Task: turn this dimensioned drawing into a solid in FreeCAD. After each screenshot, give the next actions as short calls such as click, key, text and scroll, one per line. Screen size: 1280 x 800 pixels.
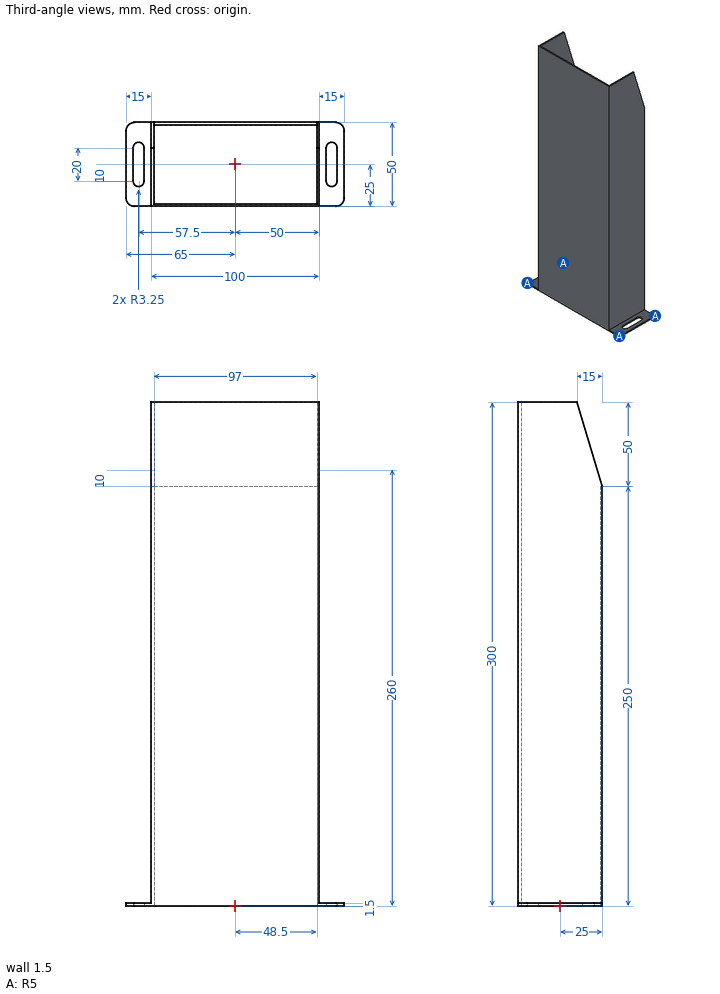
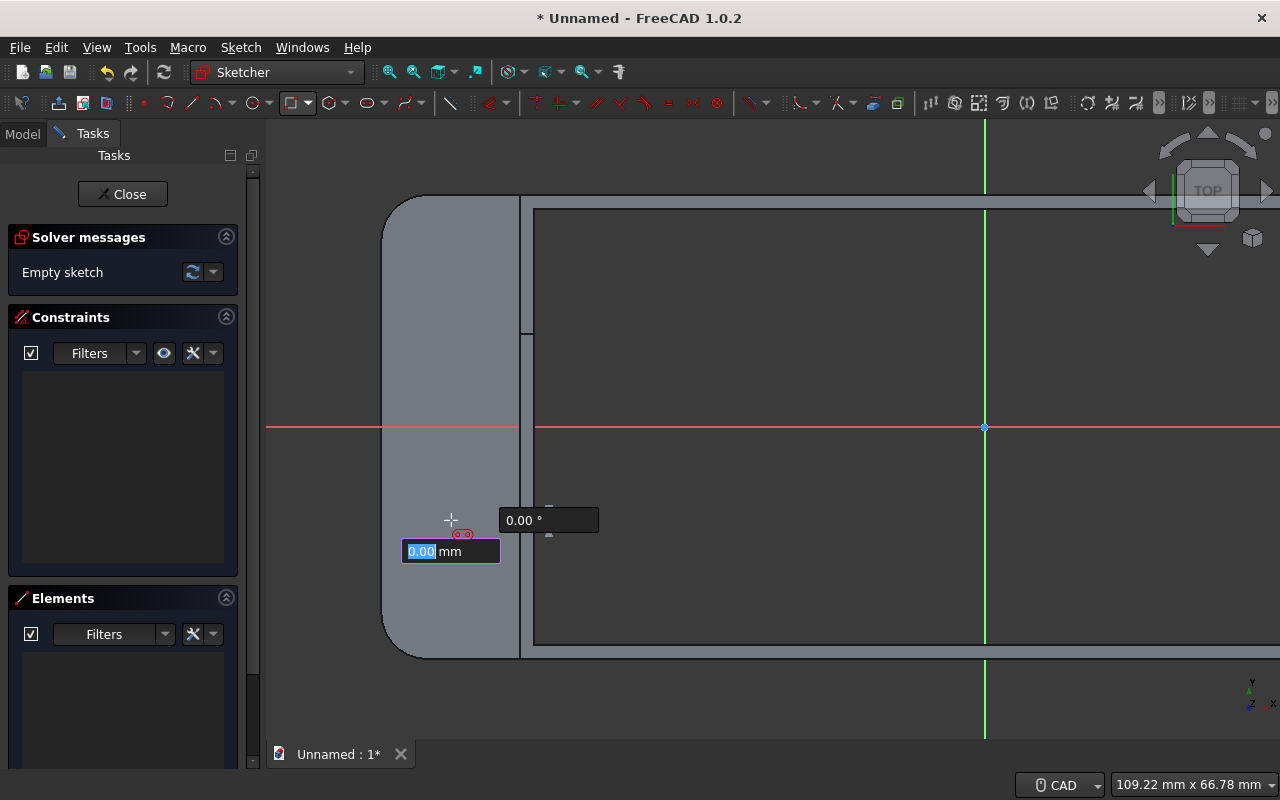
click(451, 334)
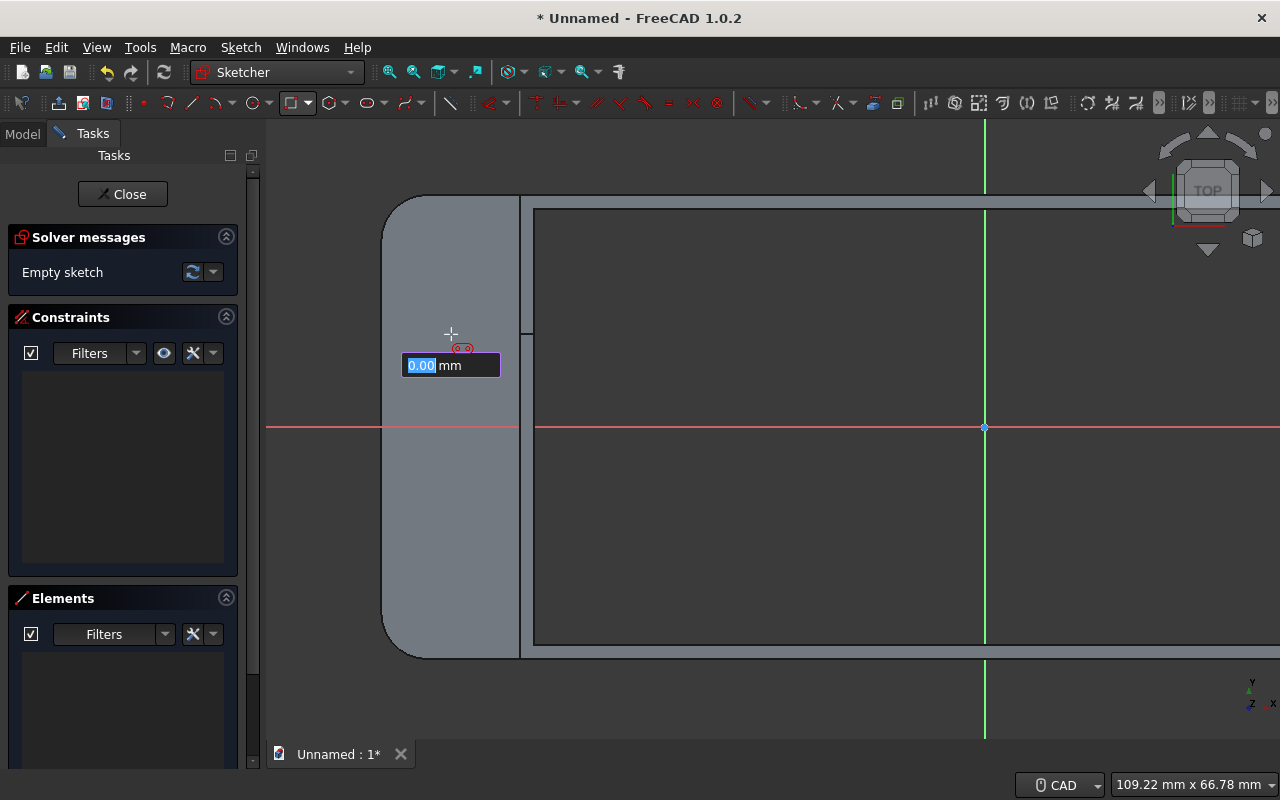
click(421, 399)
key(Escape)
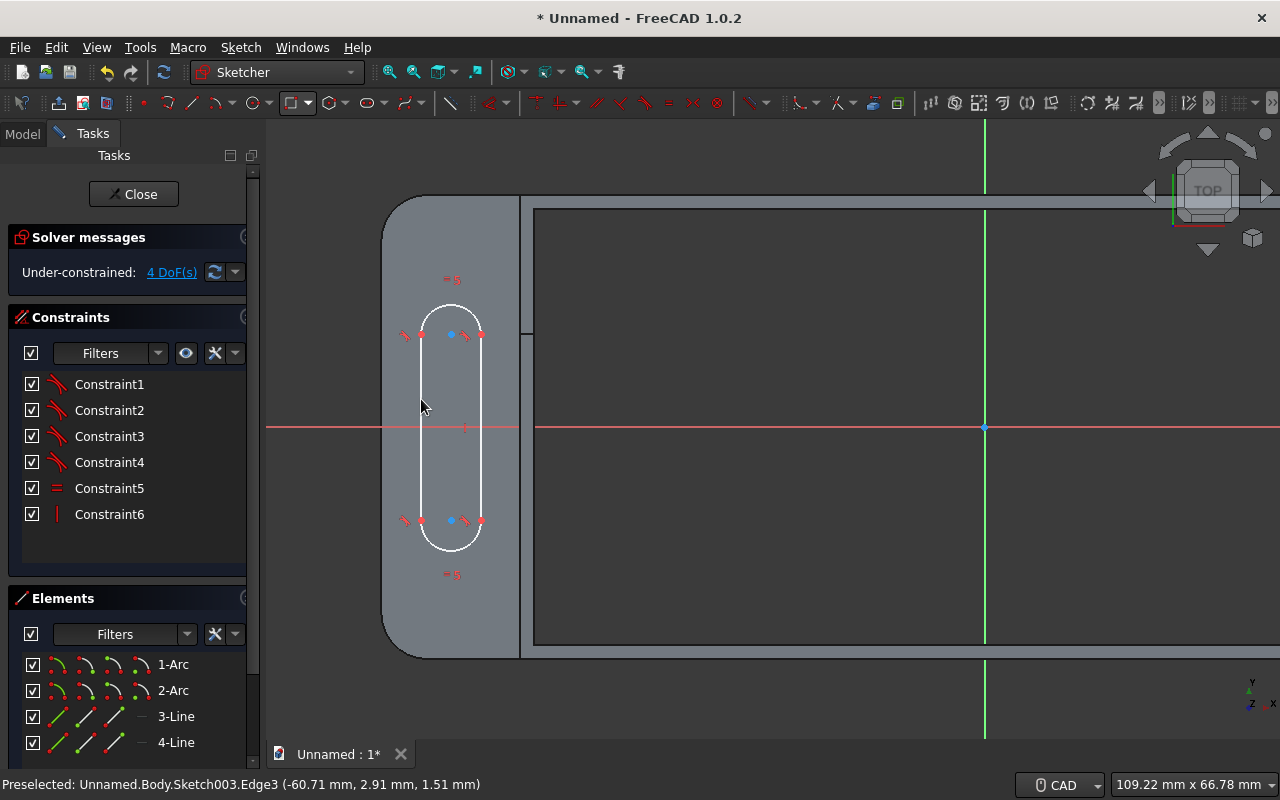
click(490, 104)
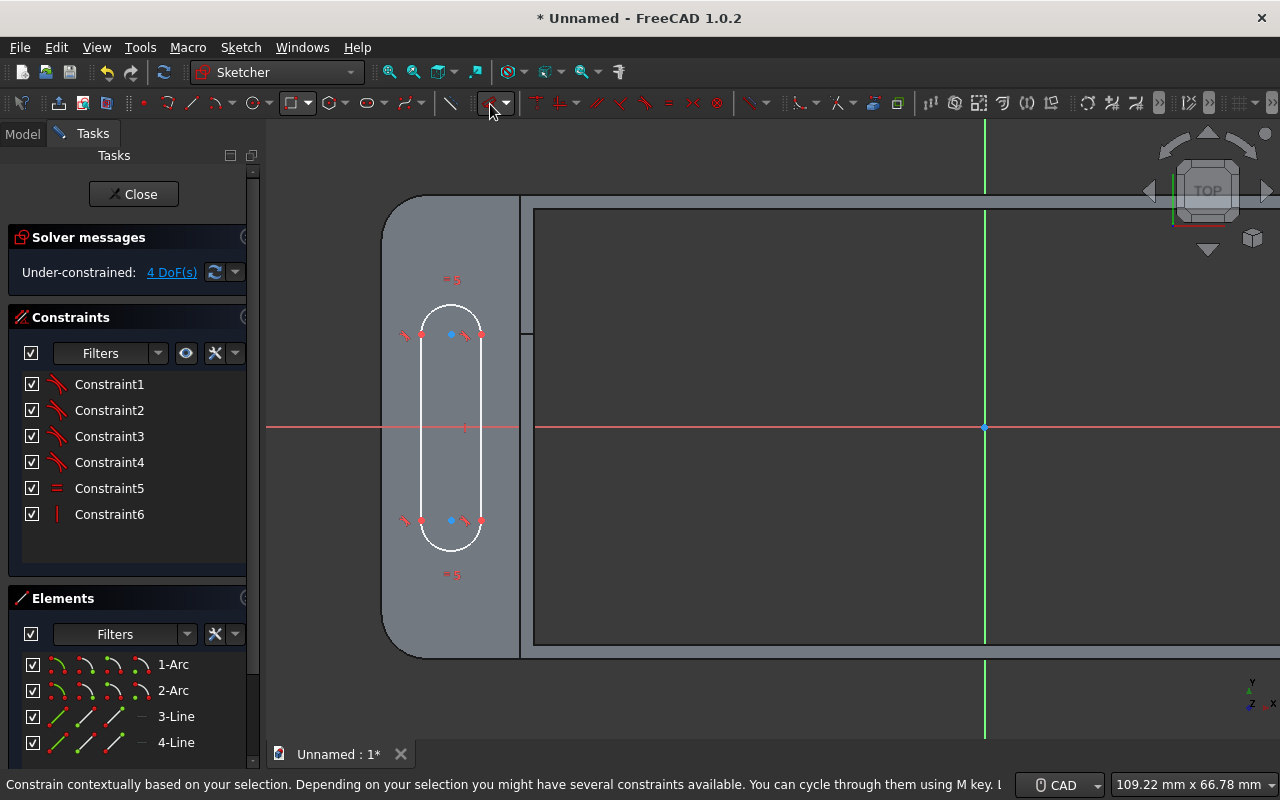
scroll(433, 545, up, 2)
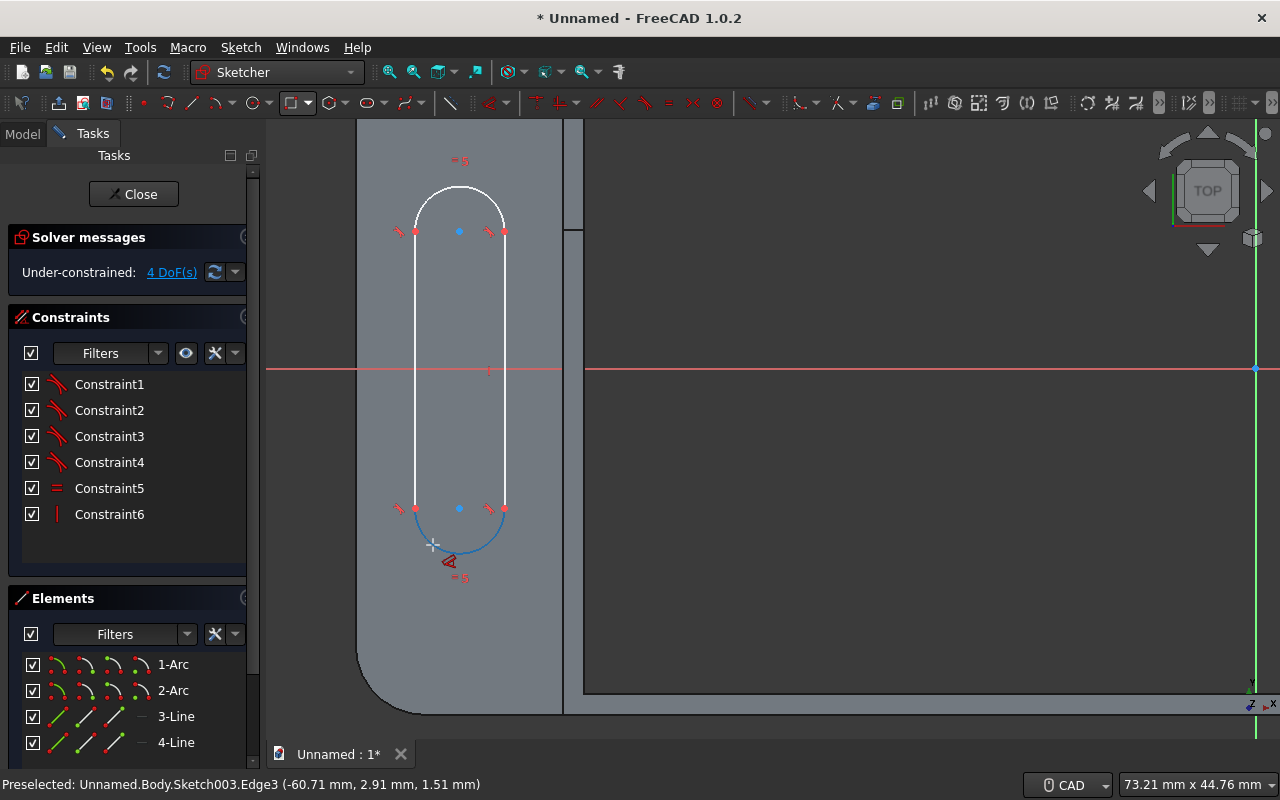
click(433, 545)
click(414, 571)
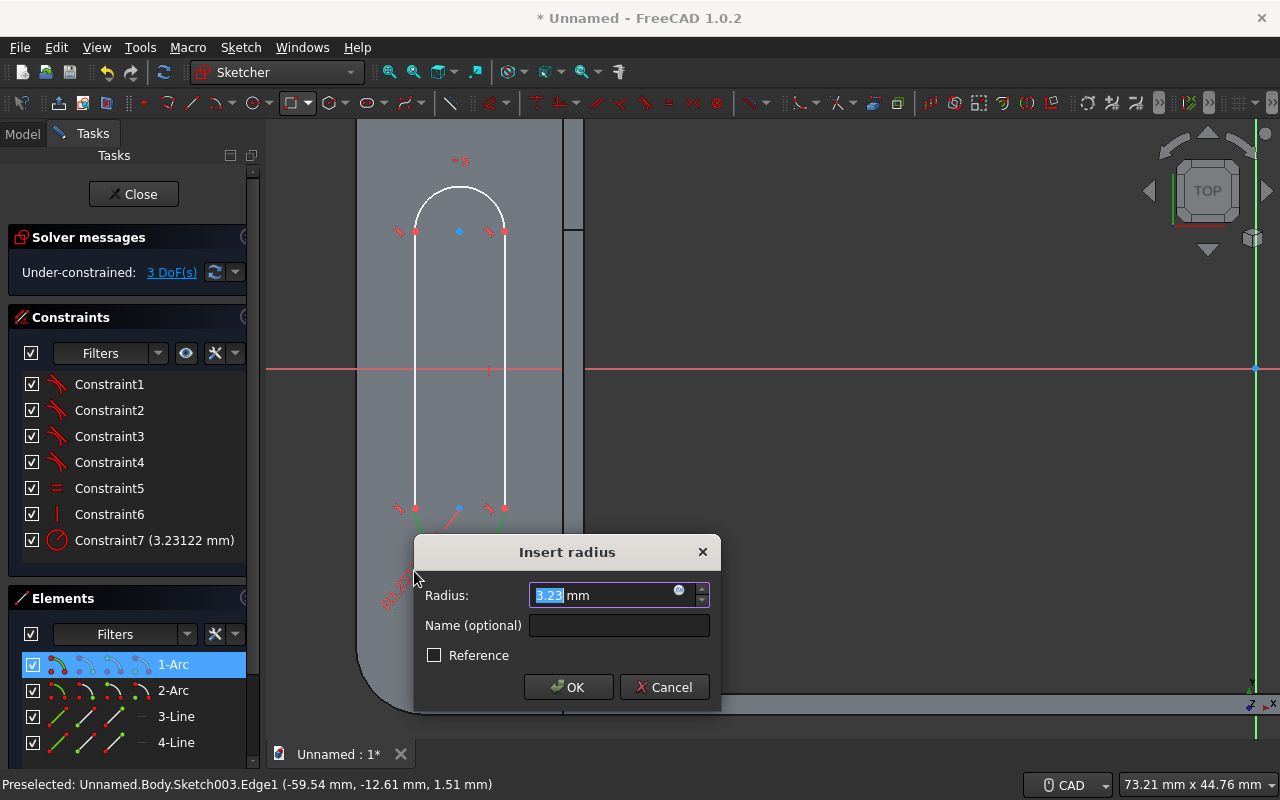
text(3.25)
key(Return)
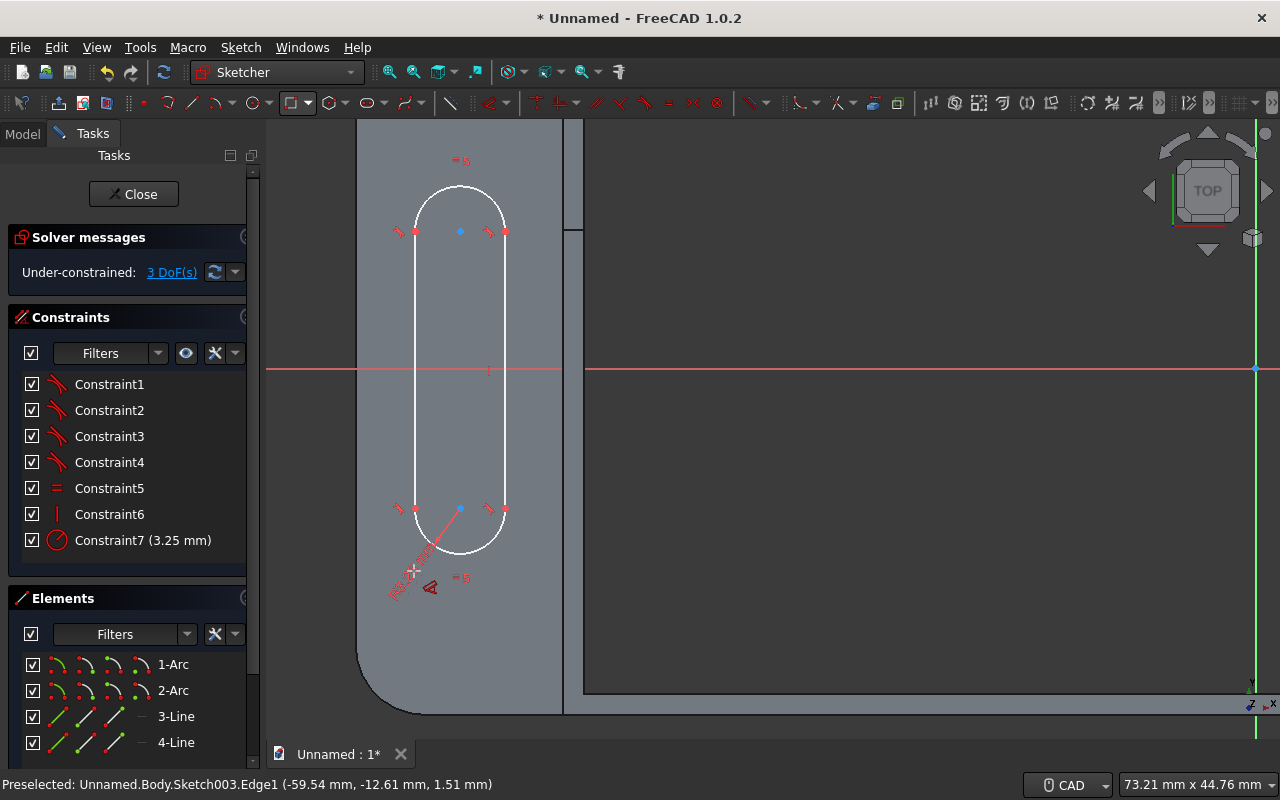
click(415, 426)
click(381, 306)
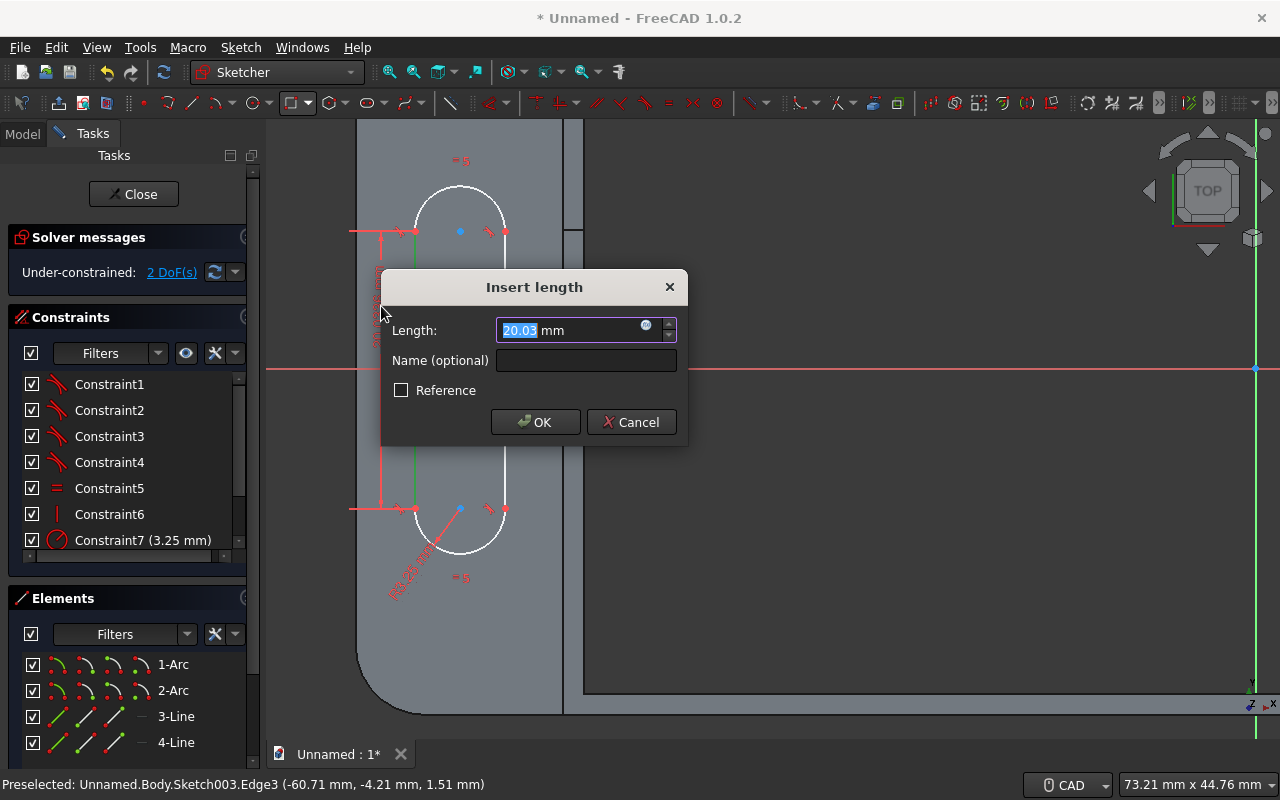
text(20)
key(Return)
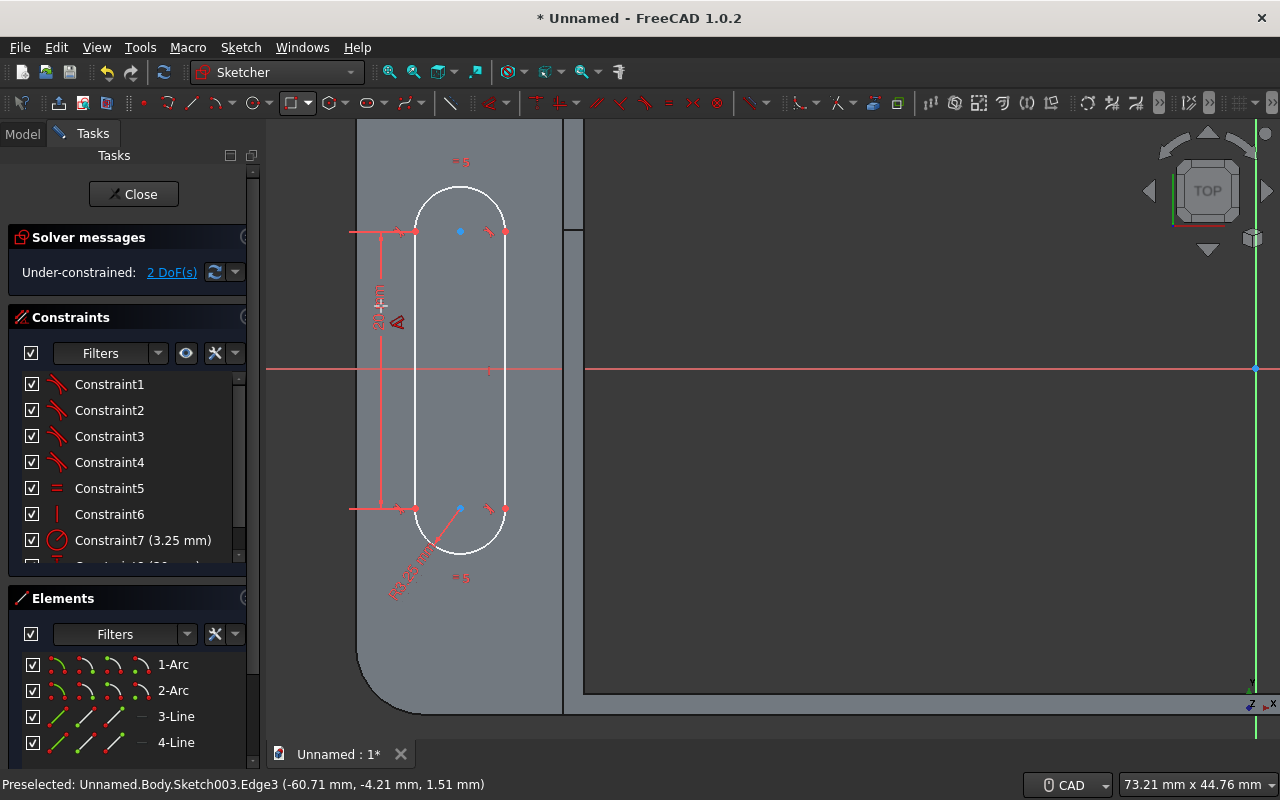
click(415, 509)
click(381, 439)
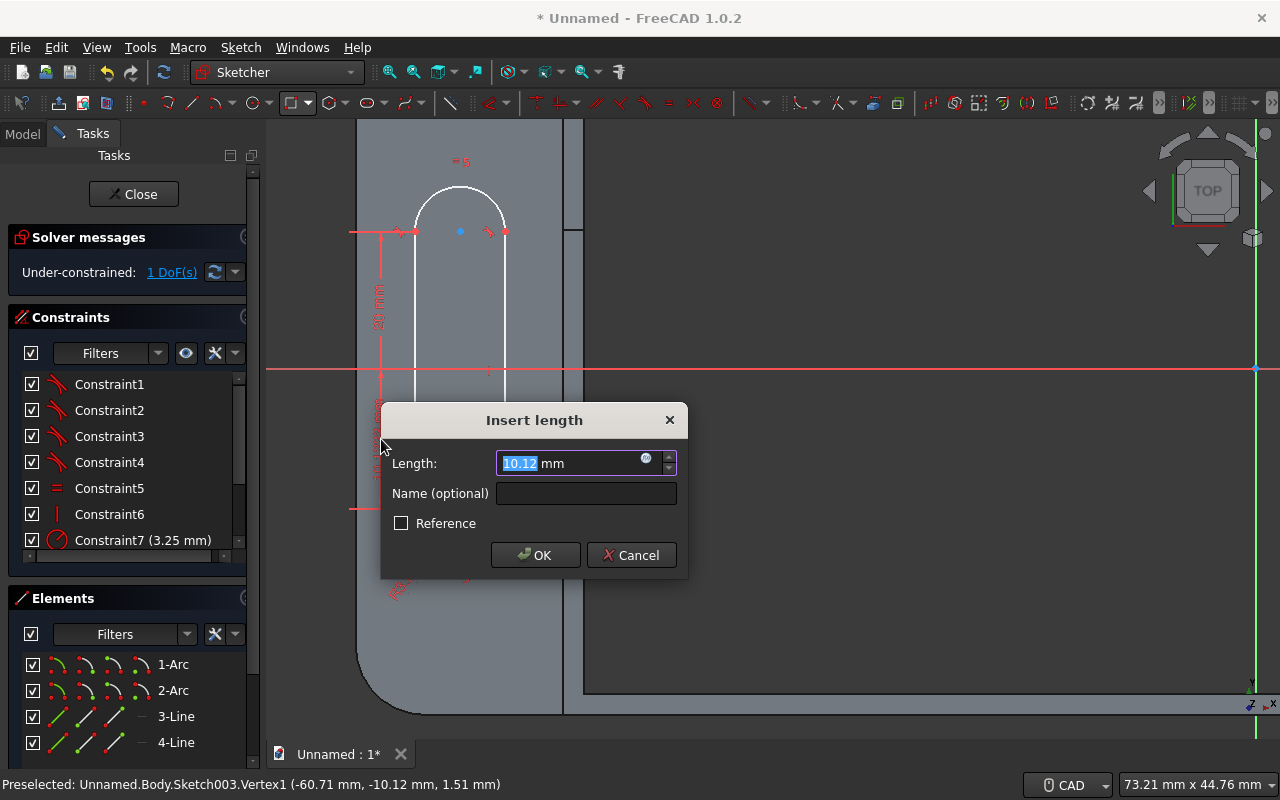
text(10)
key(Return)